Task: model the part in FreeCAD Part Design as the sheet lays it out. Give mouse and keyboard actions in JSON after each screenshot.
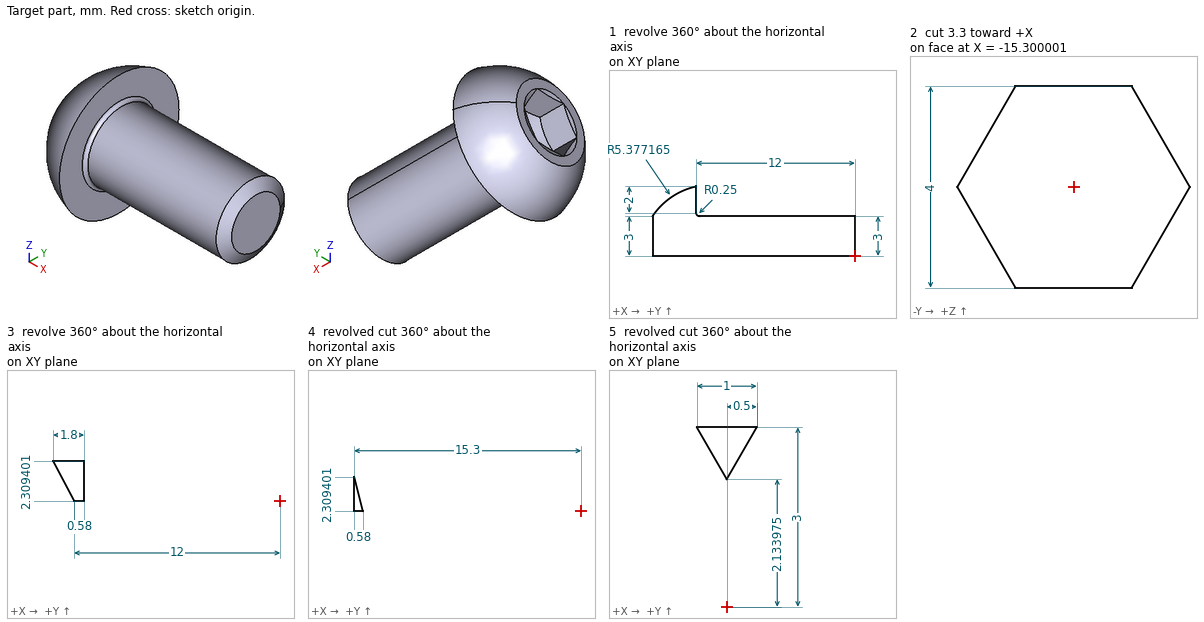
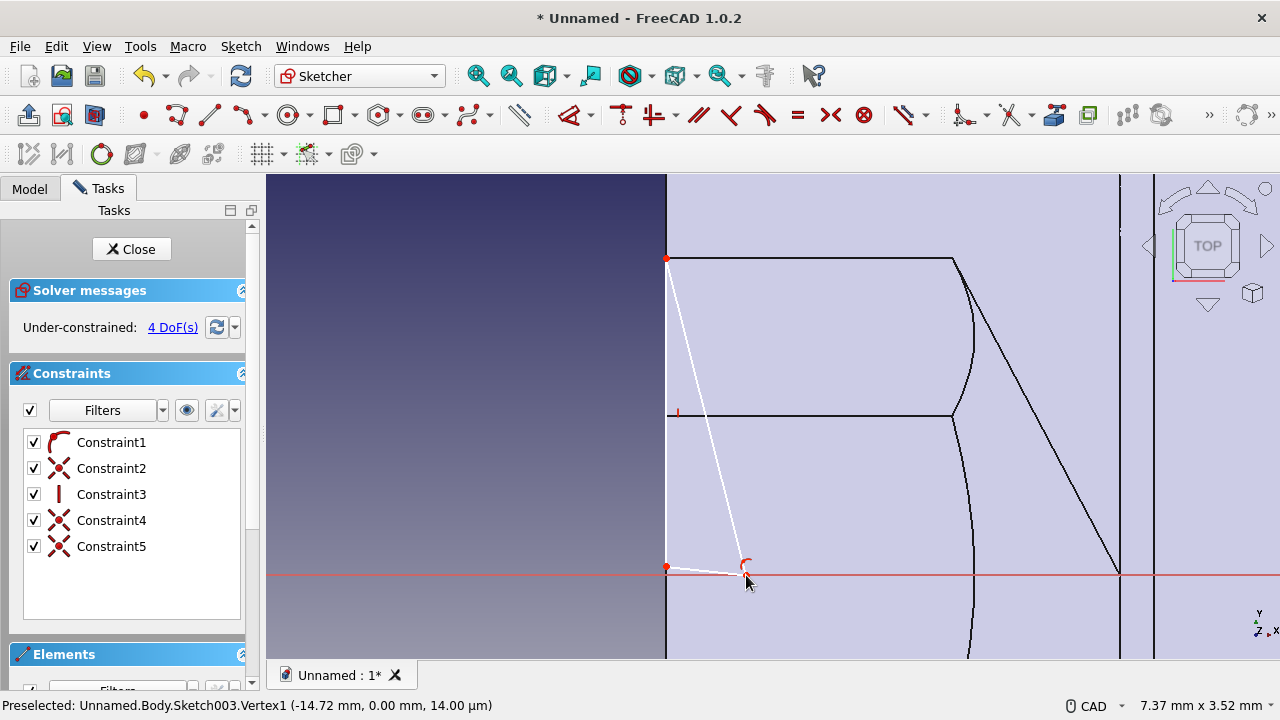
{"action": "left_click", "coordinate": [722, 573]}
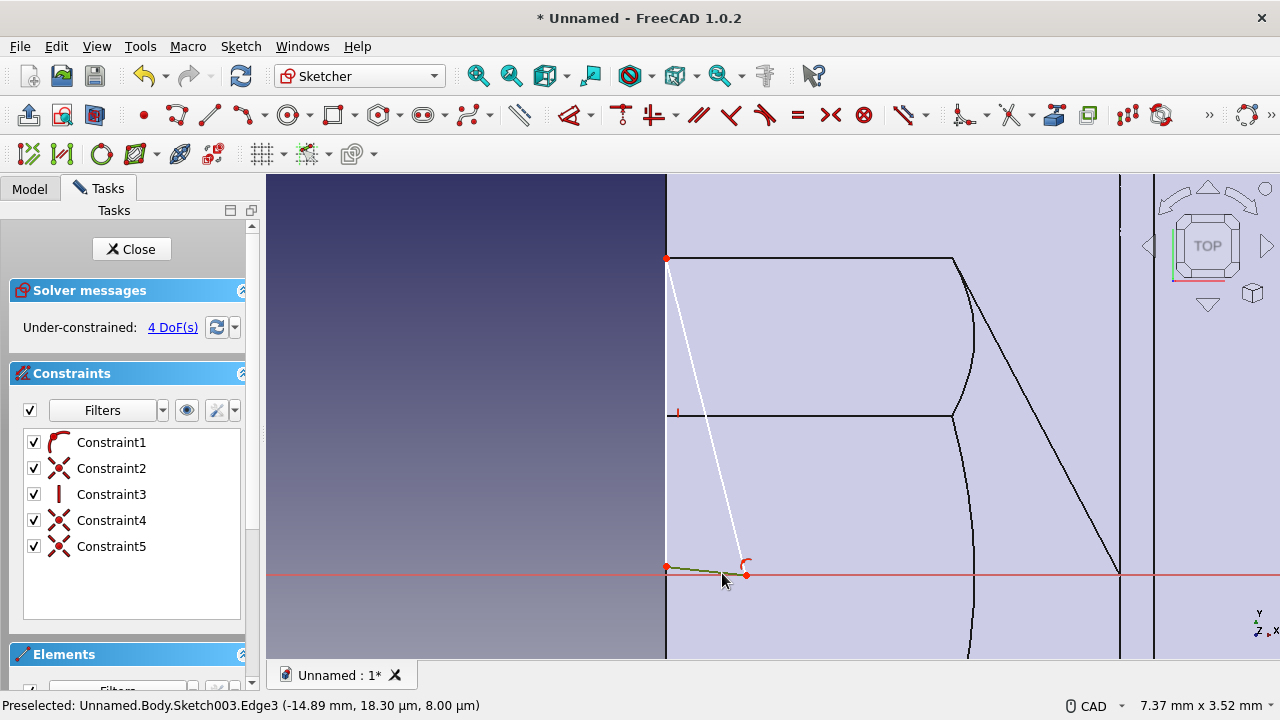
{"action": "left_click", "coordinate": [676, 116]}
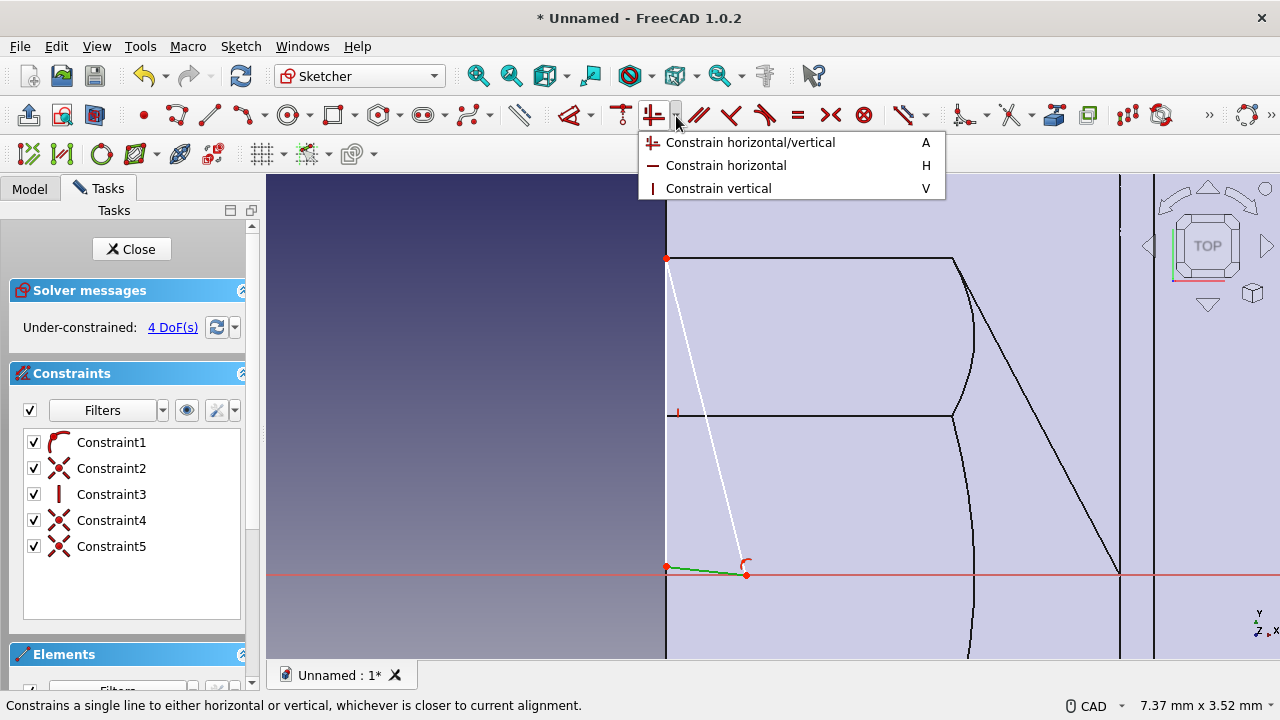
{"action": "left_click", "coordinate": [792, 166]}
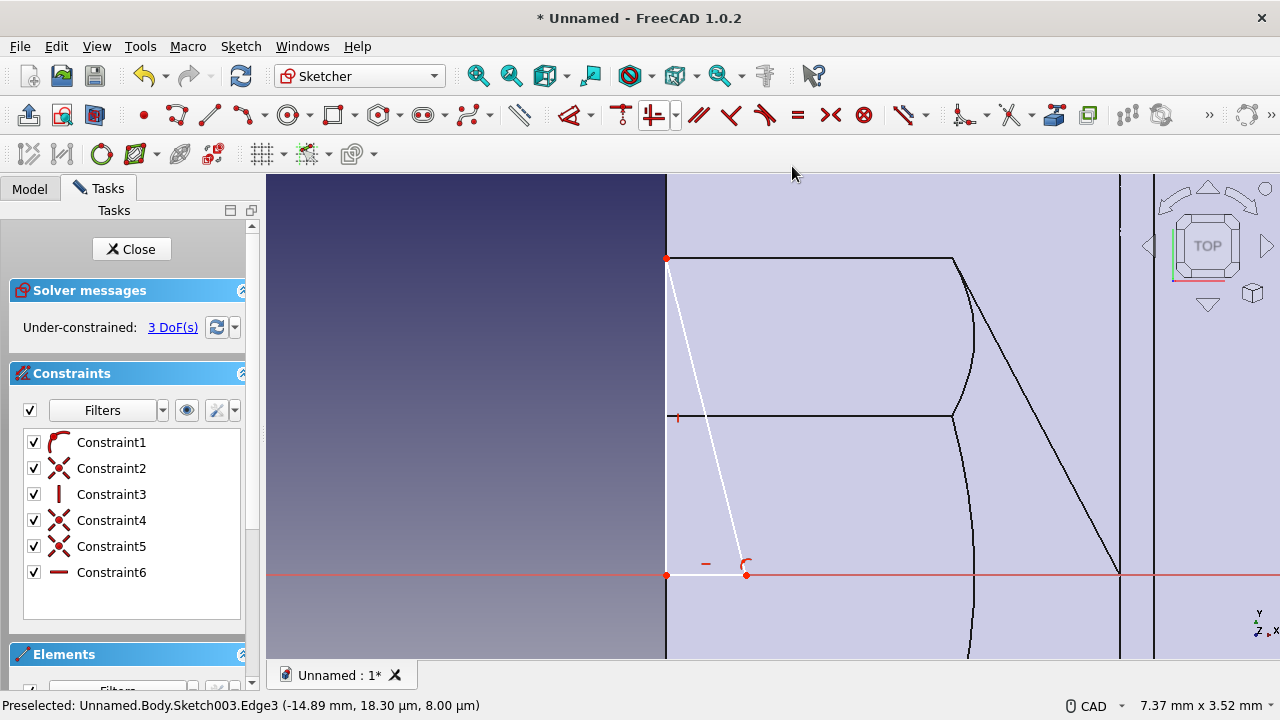
{"action": "left_click", "coordinate": [568, 116]}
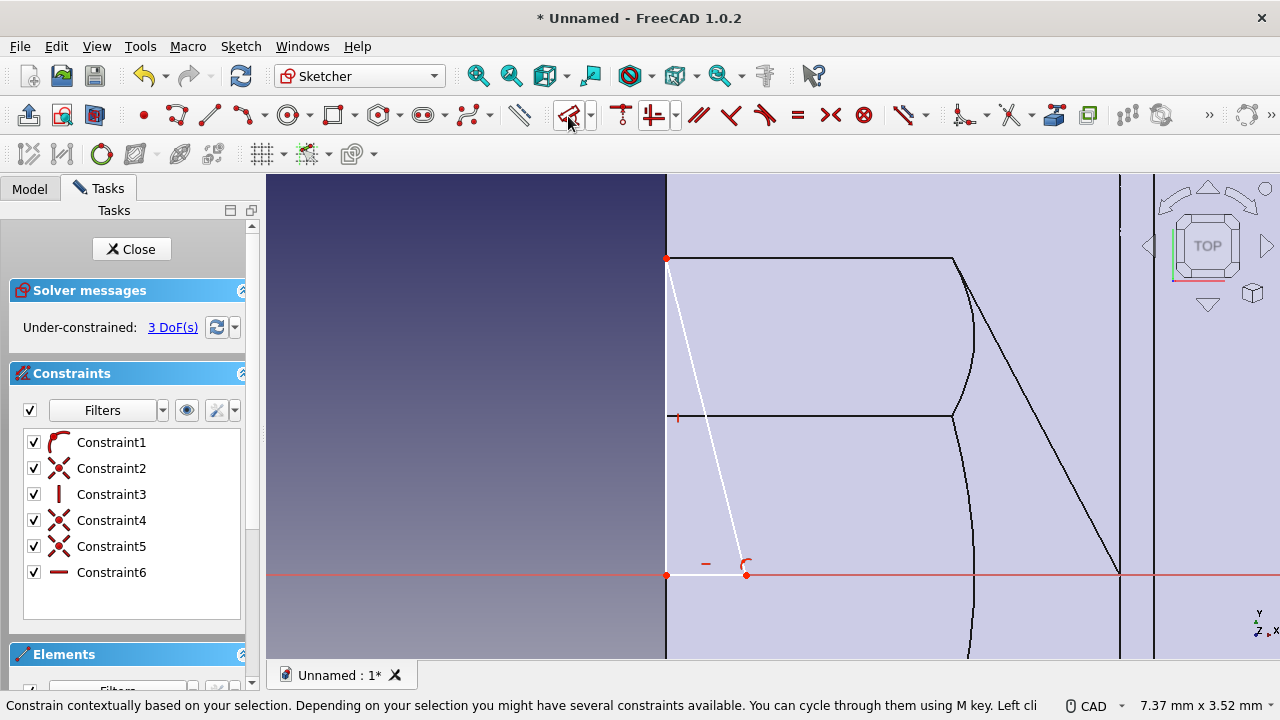
{"action": "left_click", "coordinate": [690, 575]}
{"action": "left_click", "coordinate": [706, 609]}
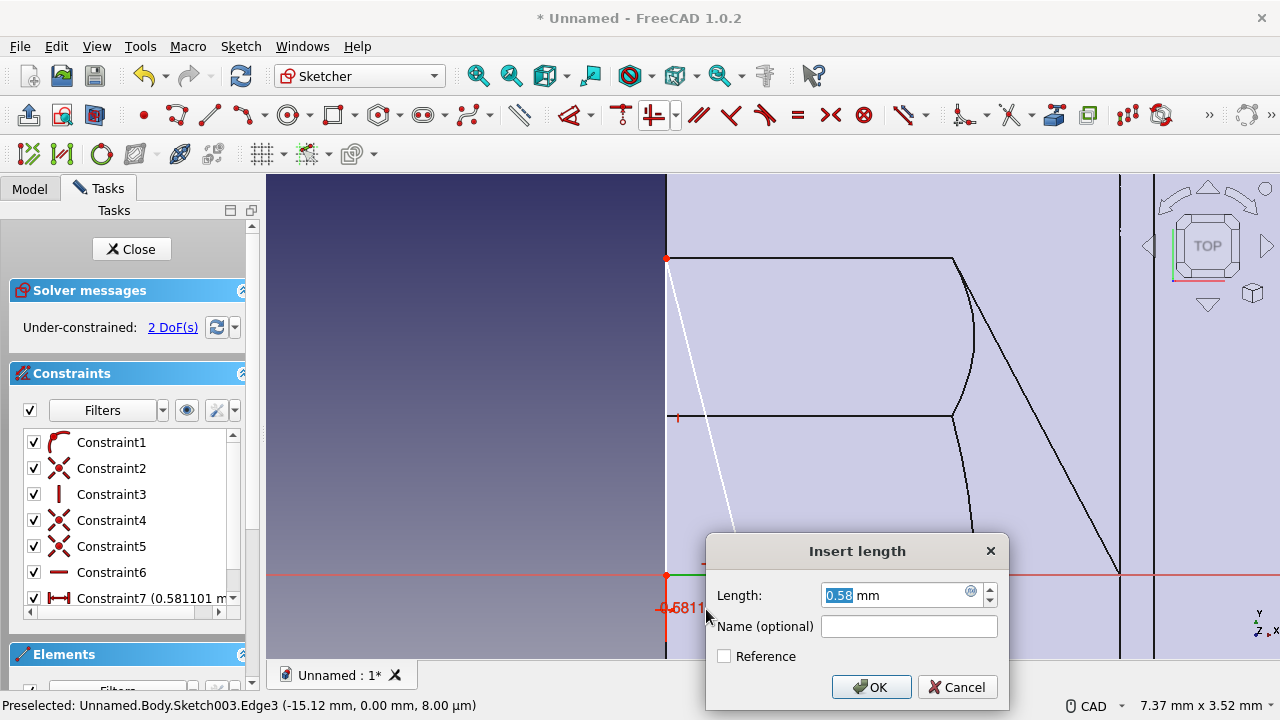
{"action": "type", "text": "0.58"}
{"action": "key", "text": "Return"}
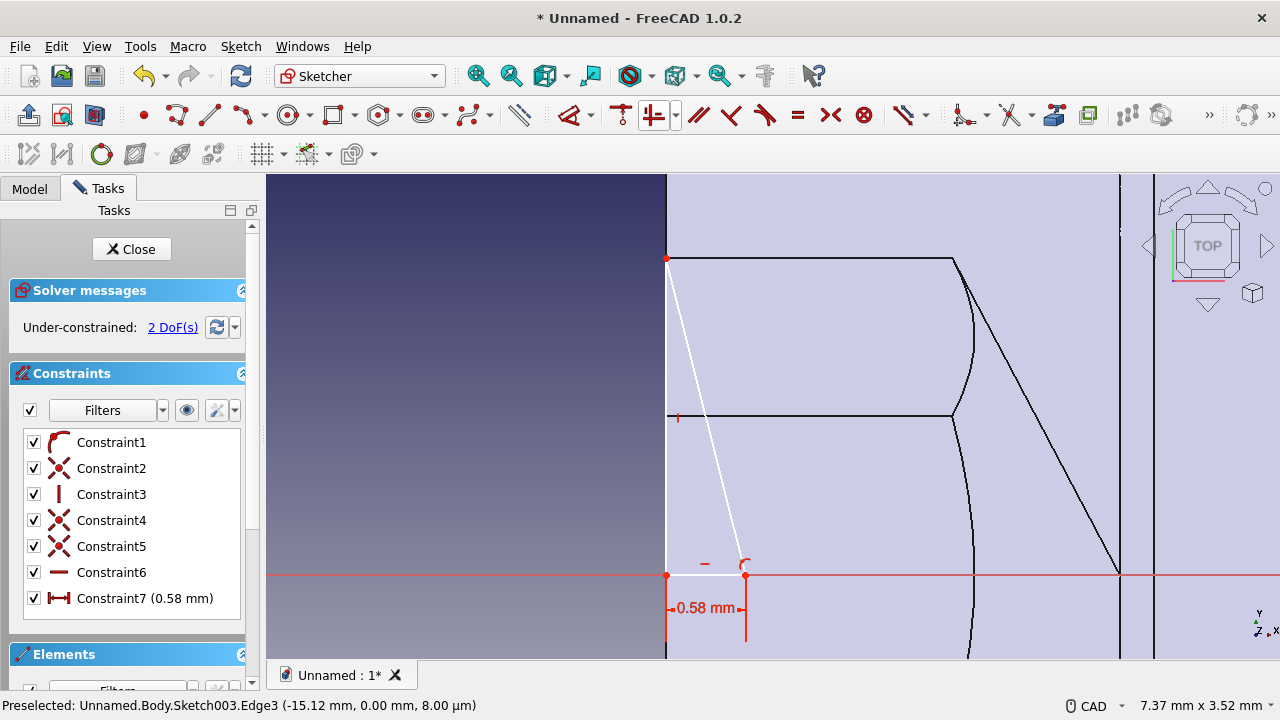
{"action": "left_click", "coordinate": [666, 259]}
{"action": "left_click", "coordinate": [891, 609]}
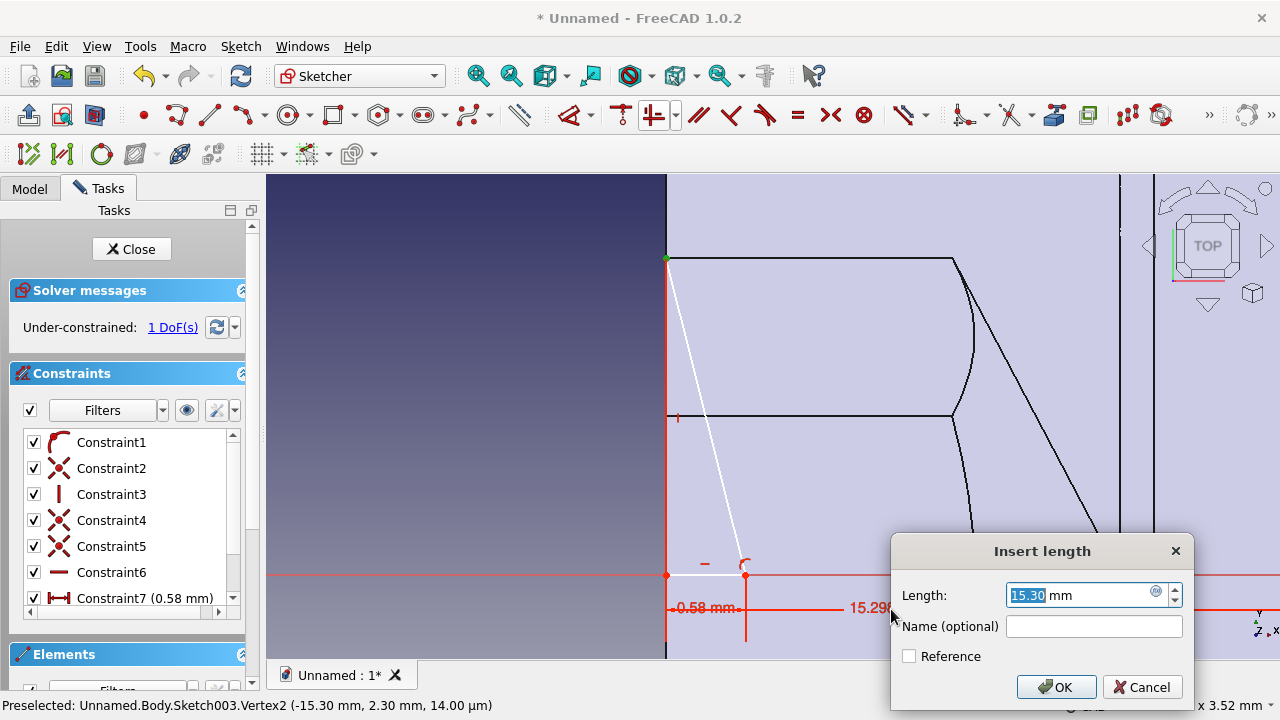
{"action": "type", "text": "15.3"}
{"action": "key", "text": "Return"}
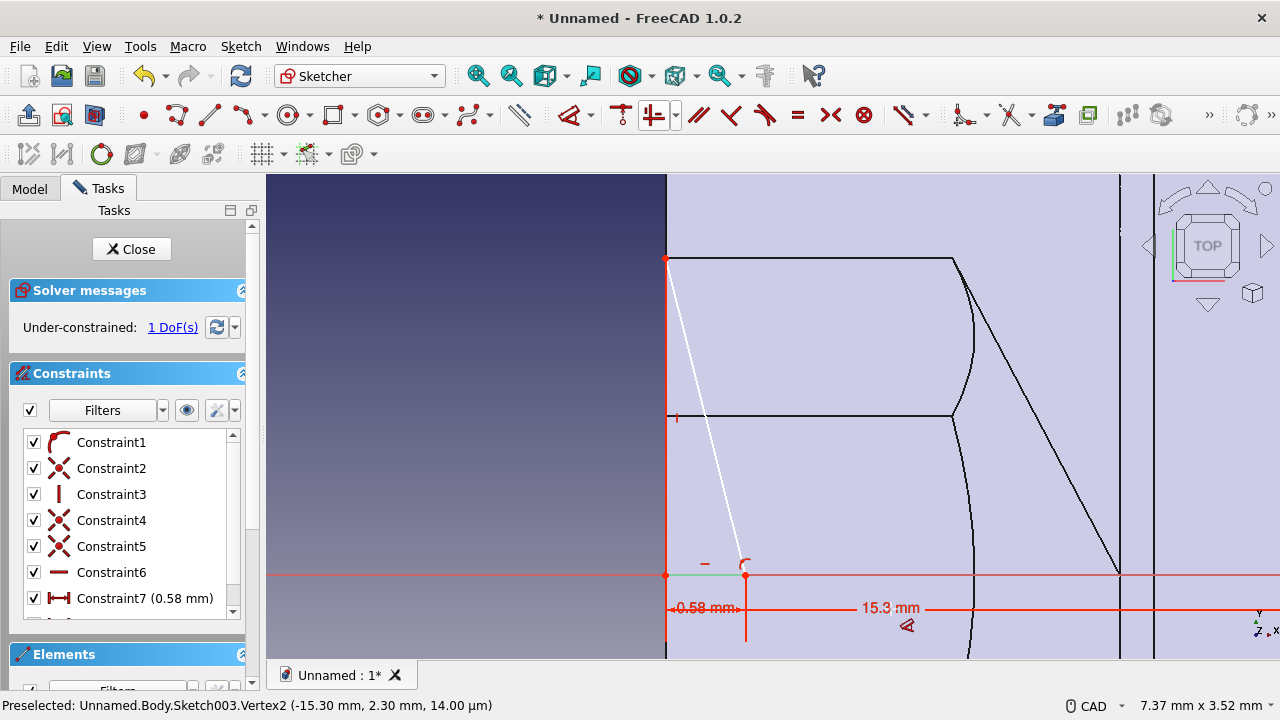
{"action": "left_click", "coordinate": [666, 354]}
{"action": "left_click", "coordinate": [632, 417]}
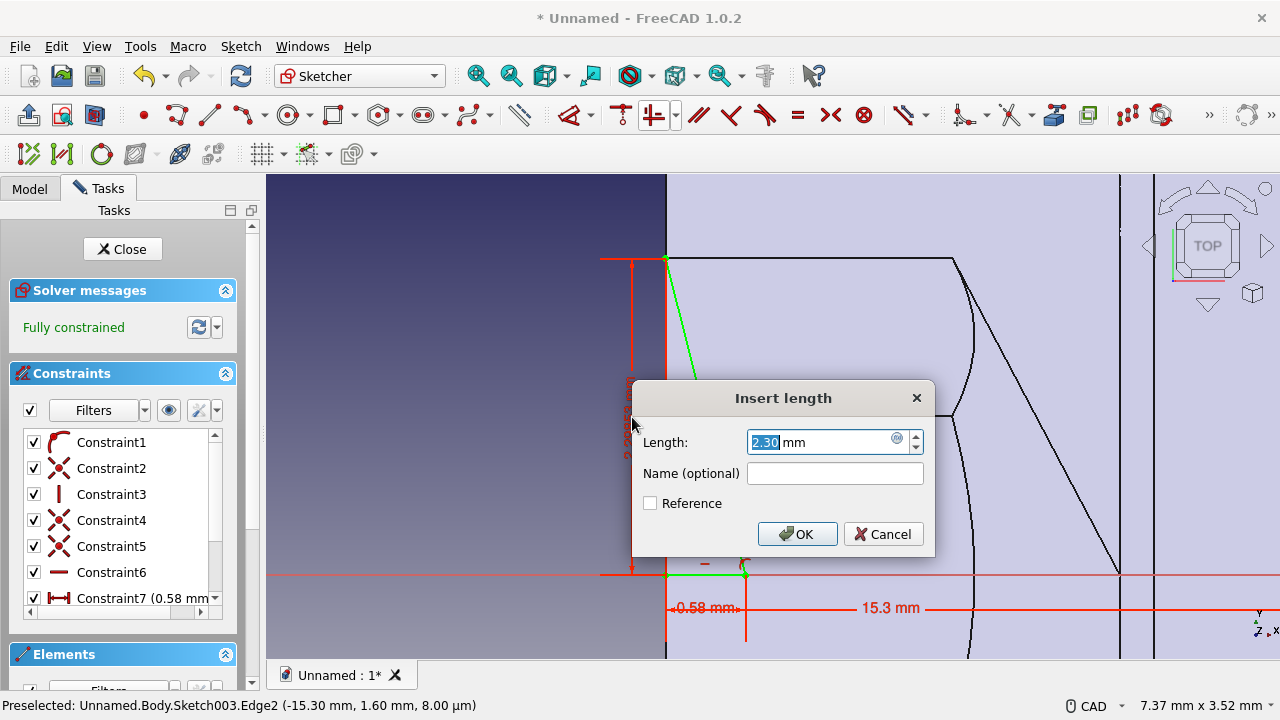
{"action": "type", "text": "2.309401"}
{"action": "key", "text": "Return"}
{"action": "key", "text": "Escape"}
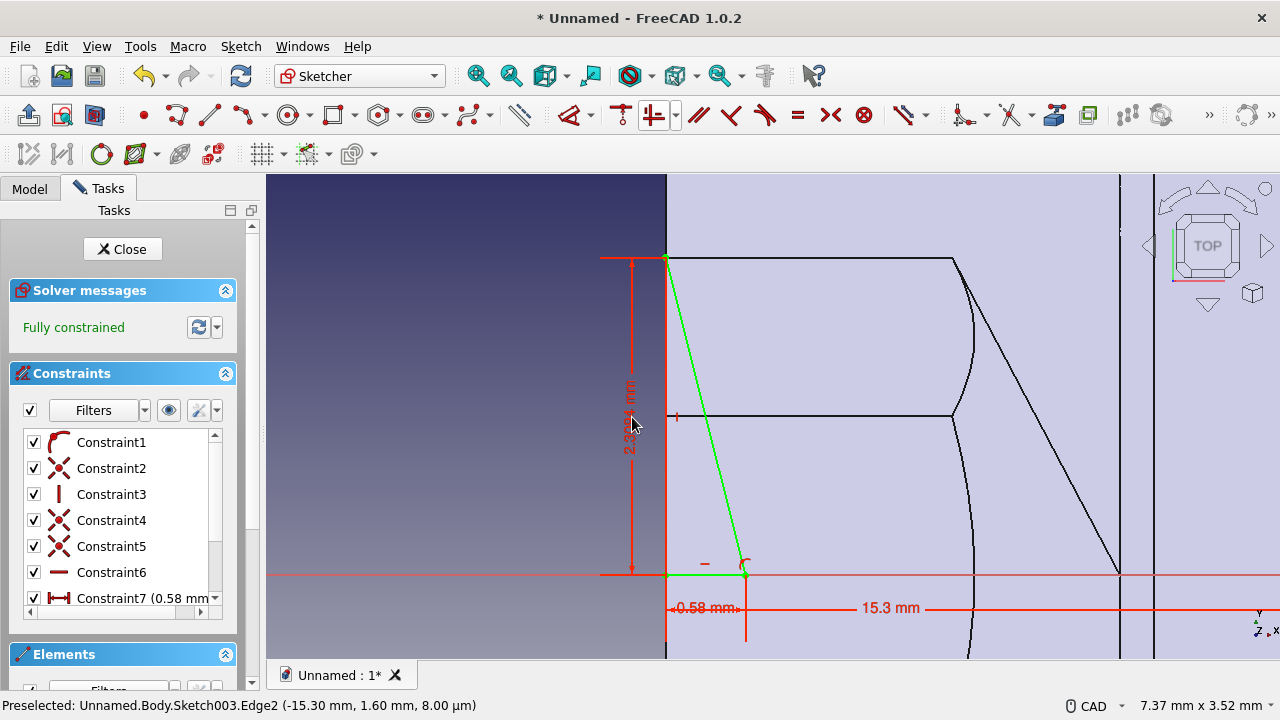
{"action": "left_click", "coordinate": [123, 249]}